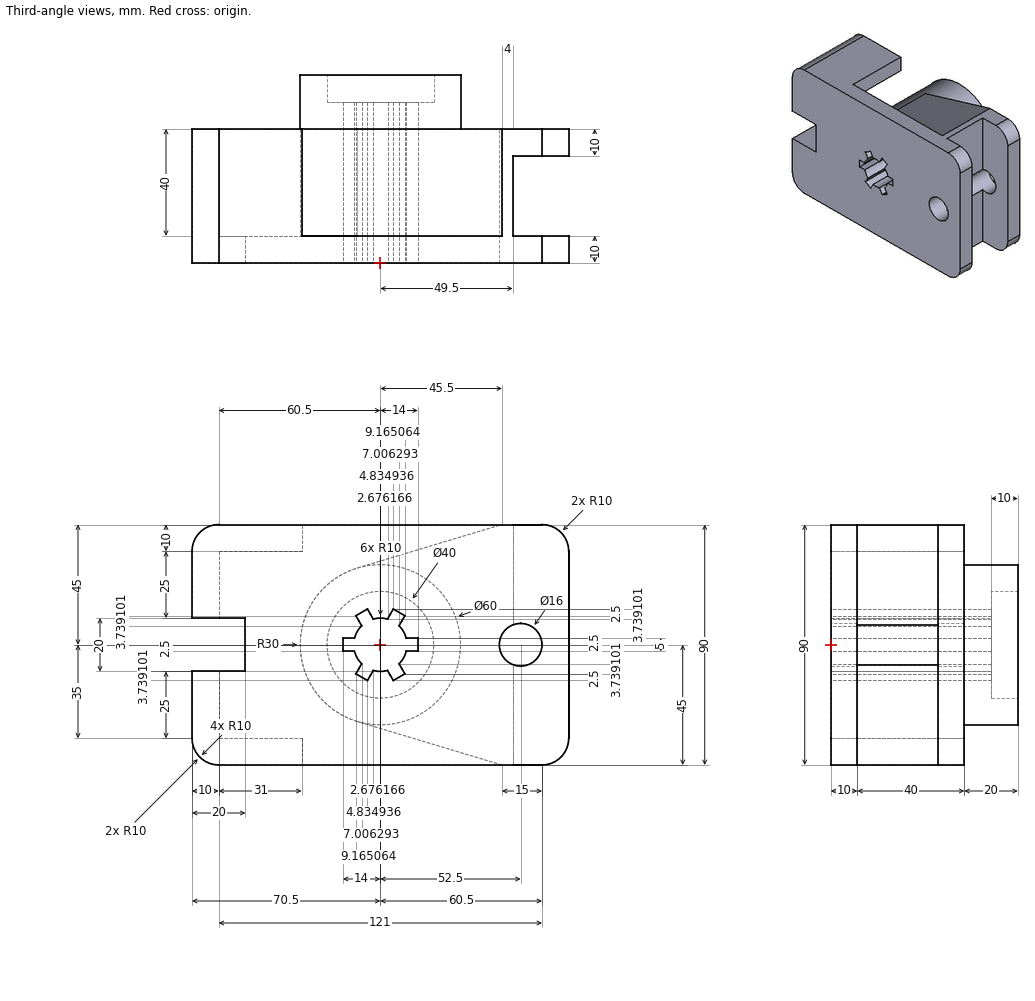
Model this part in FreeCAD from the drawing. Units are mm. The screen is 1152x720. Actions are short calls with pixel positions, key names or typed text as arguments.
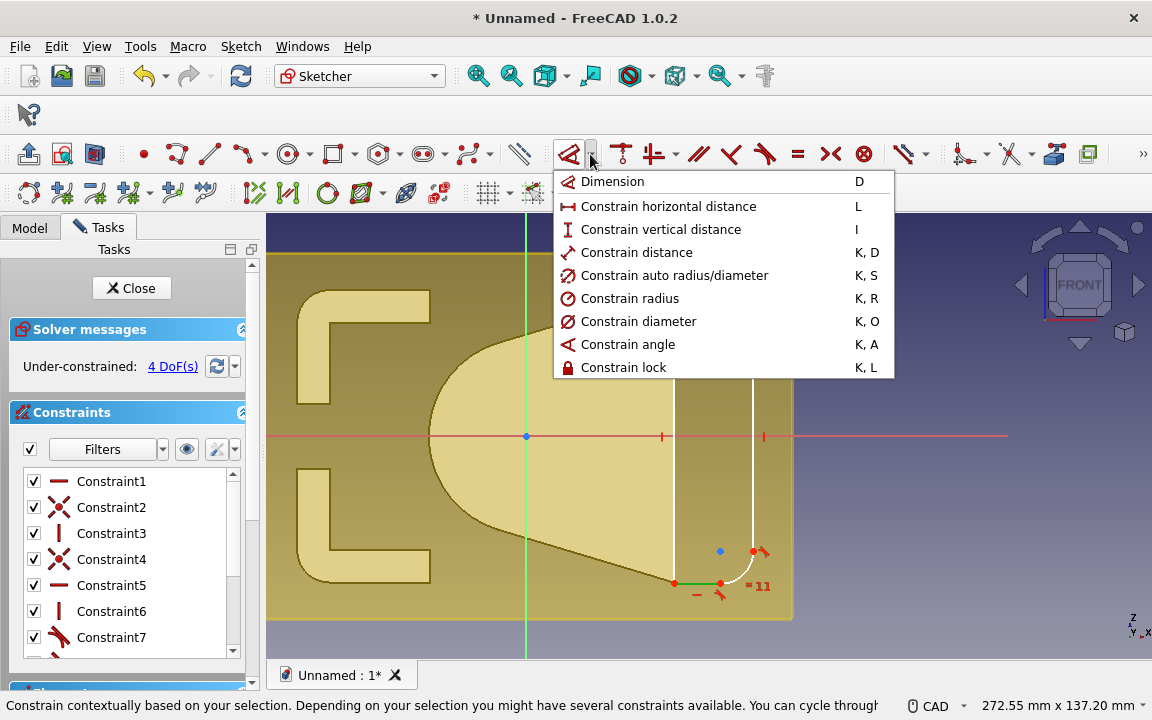
click(724, 206)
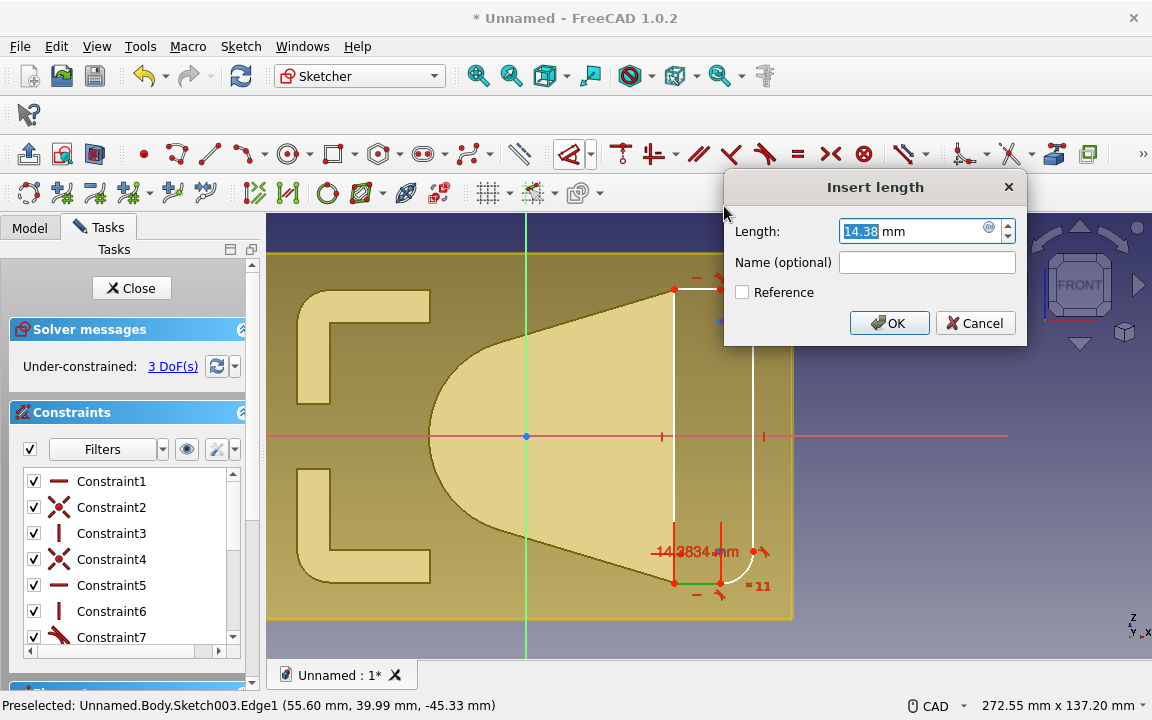
text(15)
key(Return)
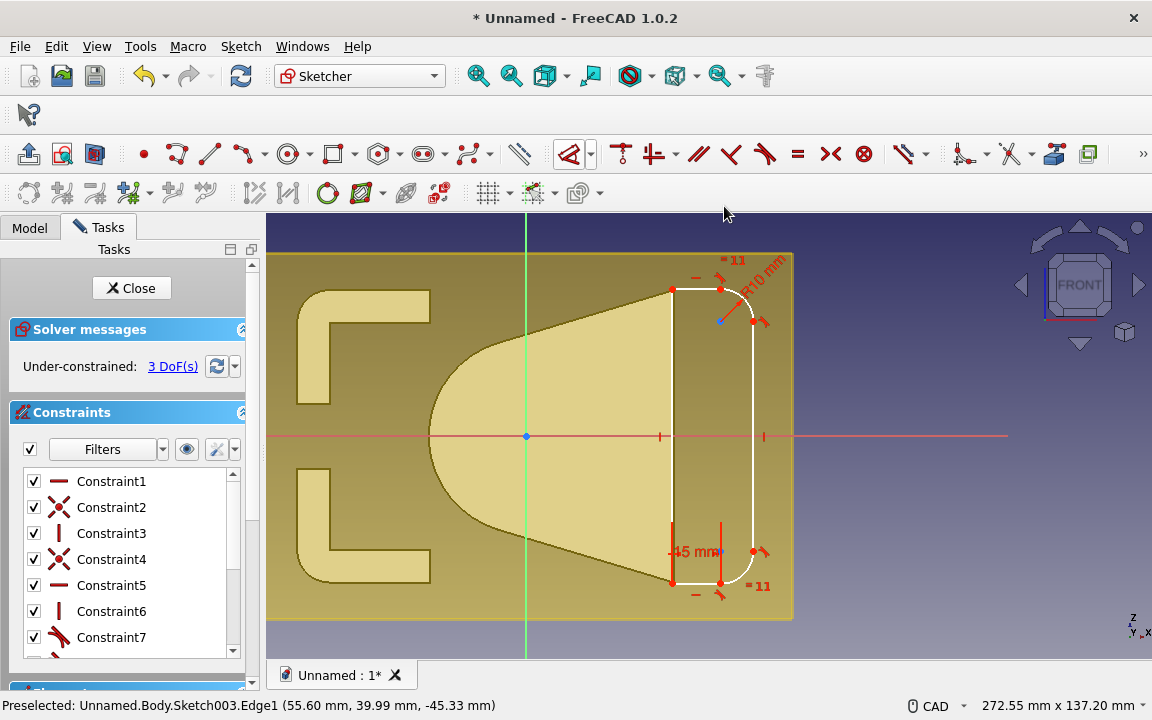
click(672, 495)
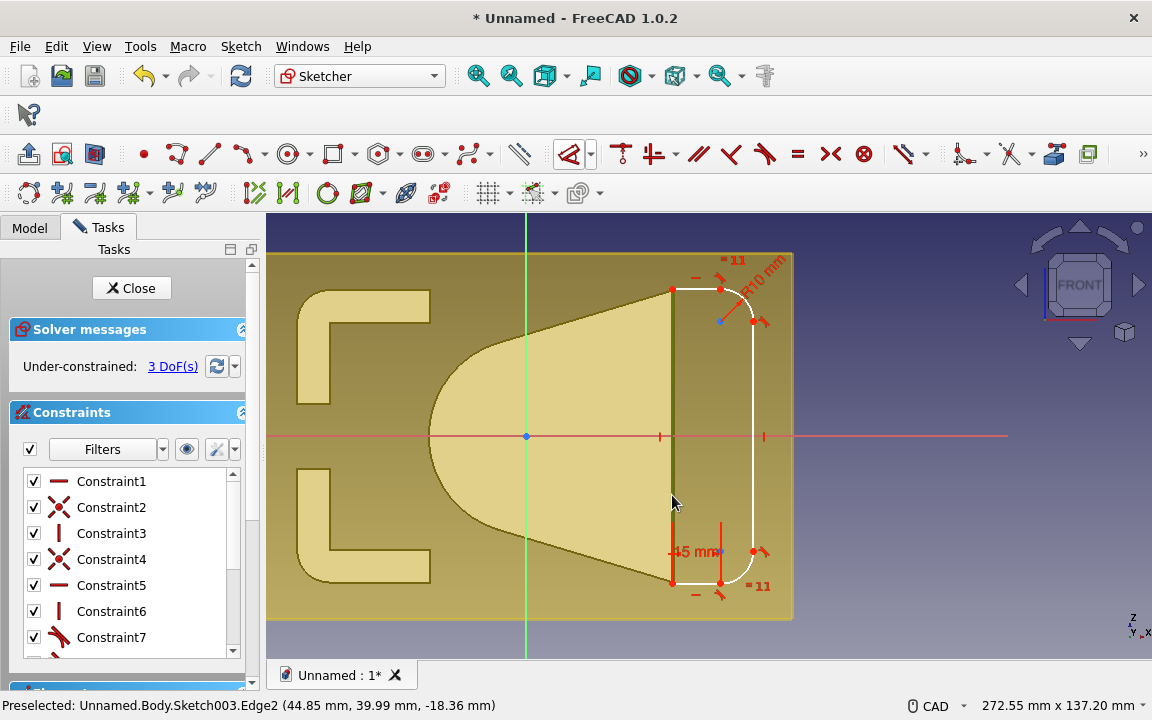
key(i)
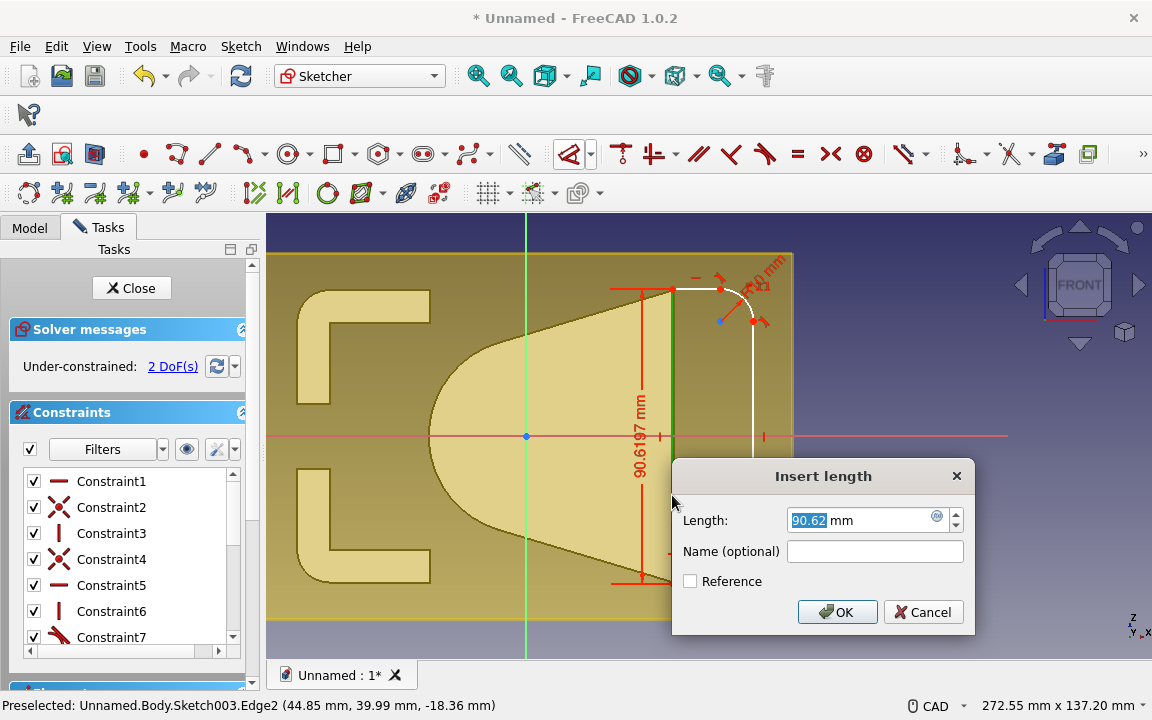
text(90)
key(Return)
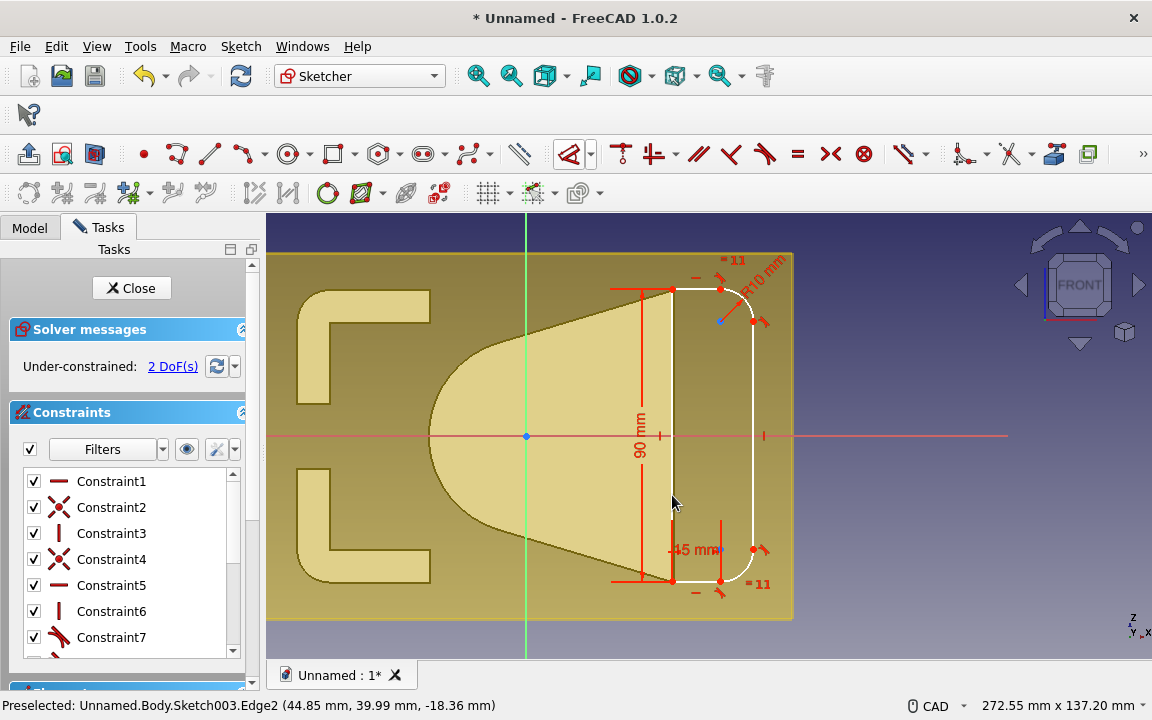
click(721, 582)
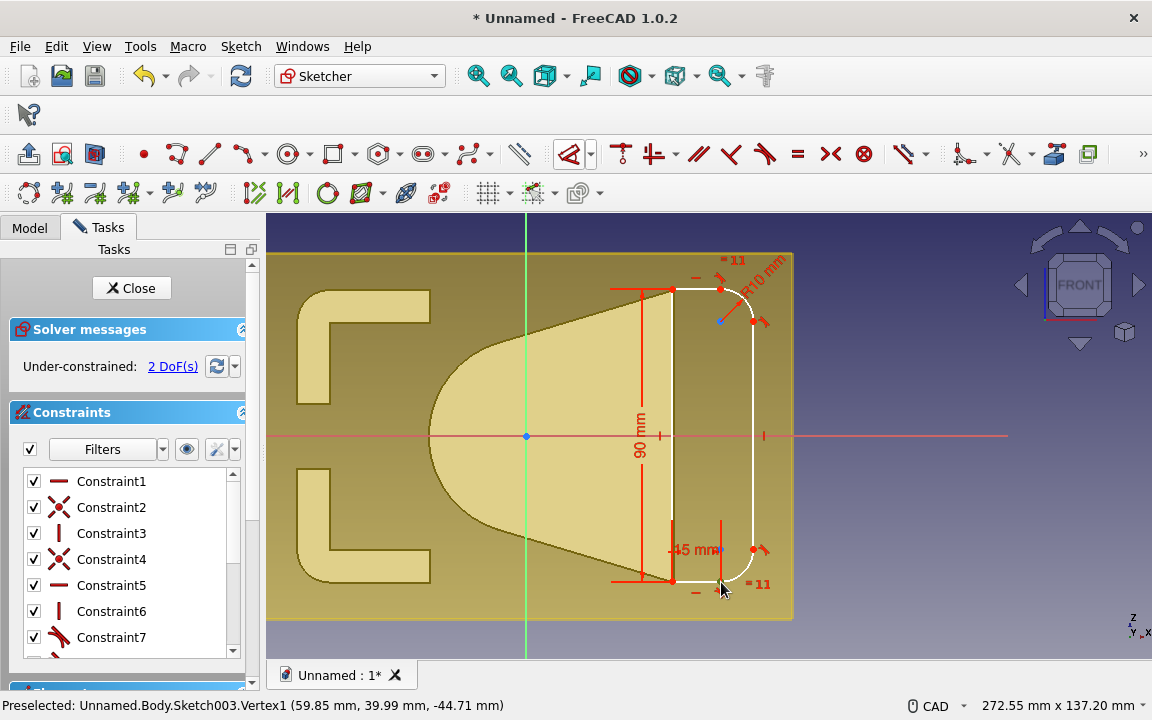
click(590, 154)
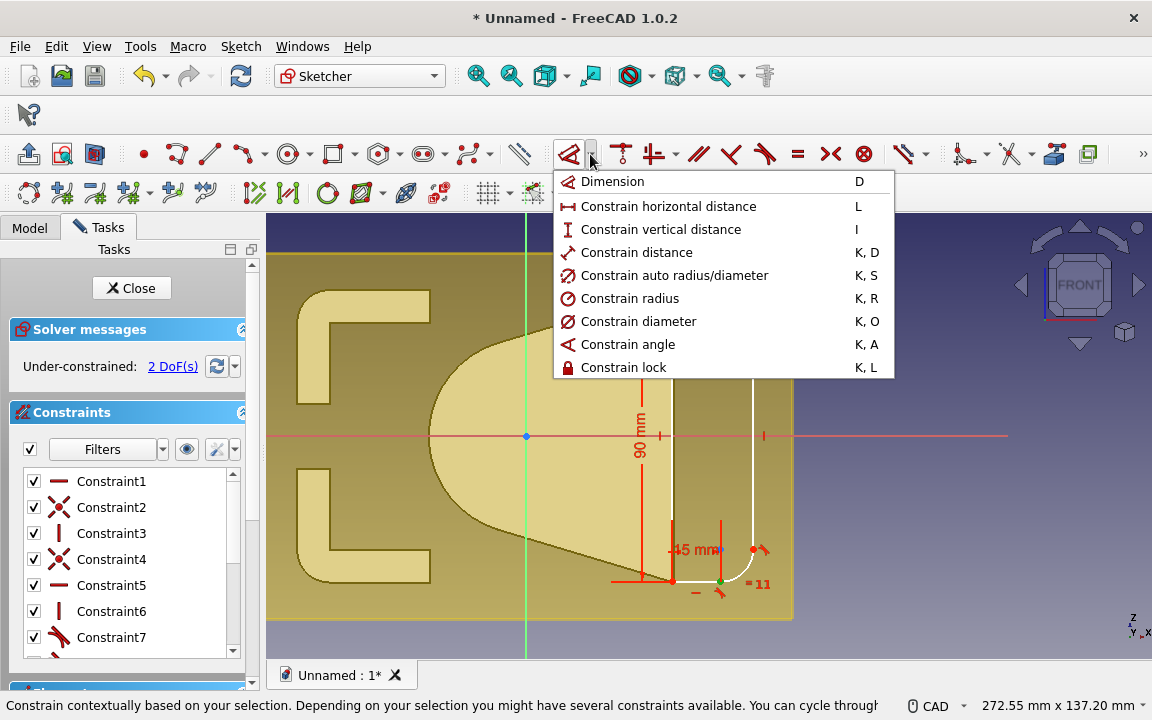
click(724, 230)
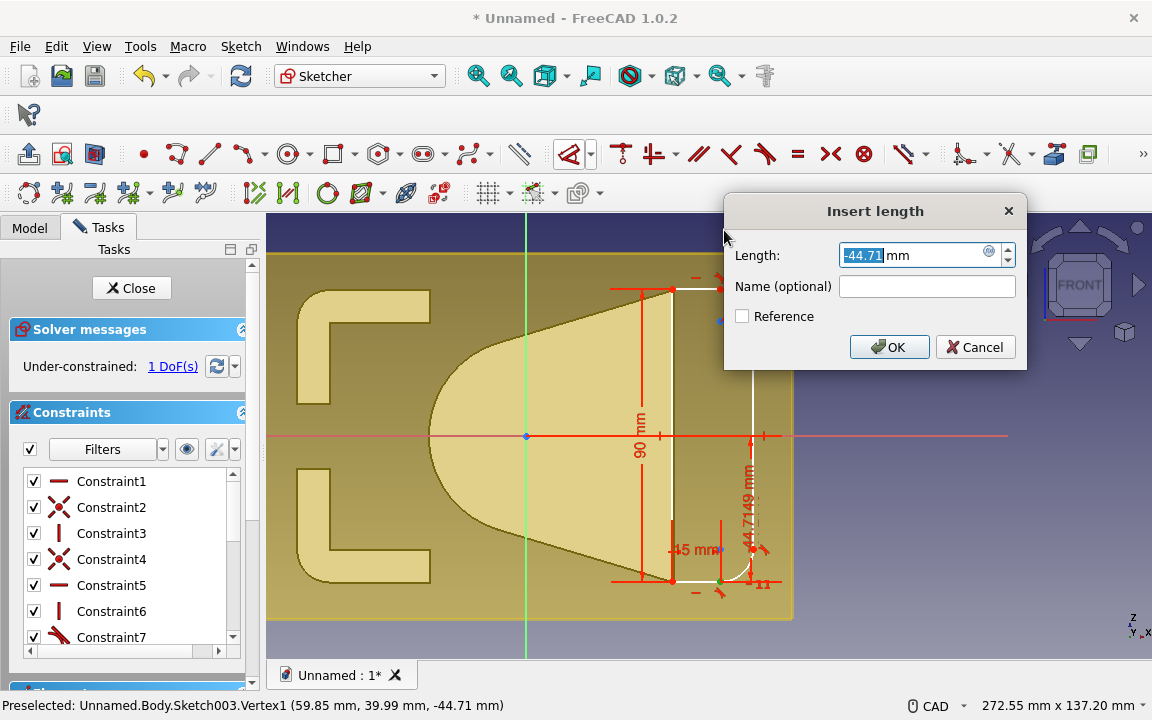
text(-45)
key(Return)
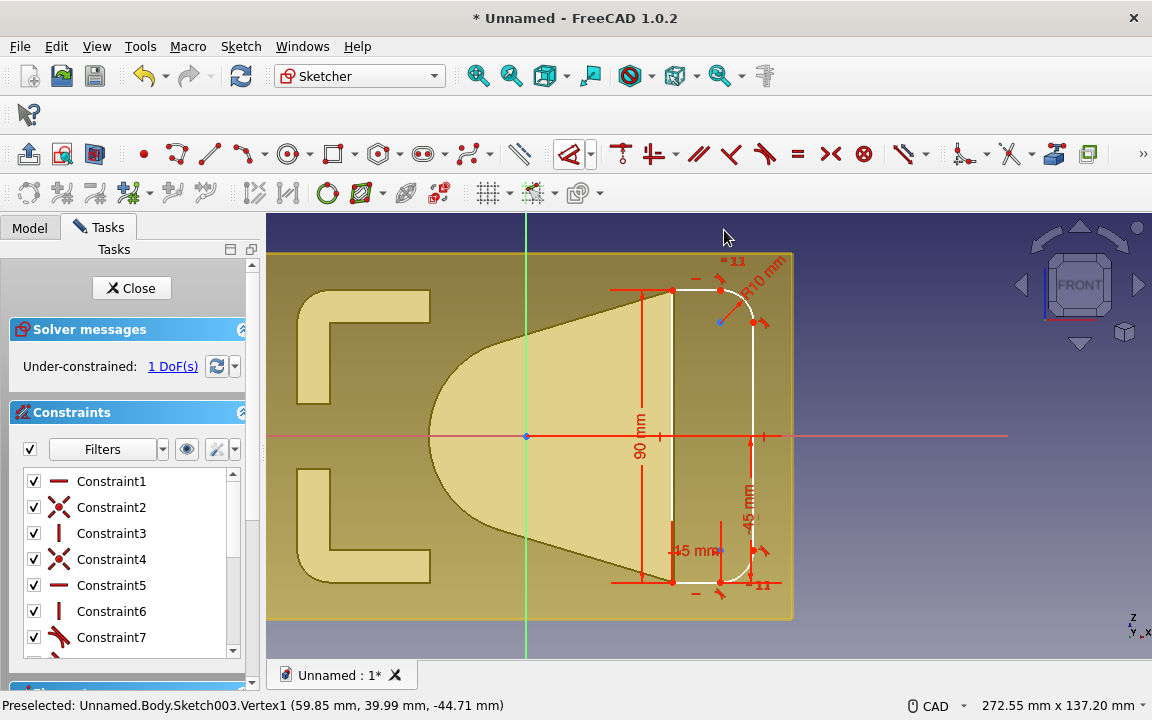
click(721, 583)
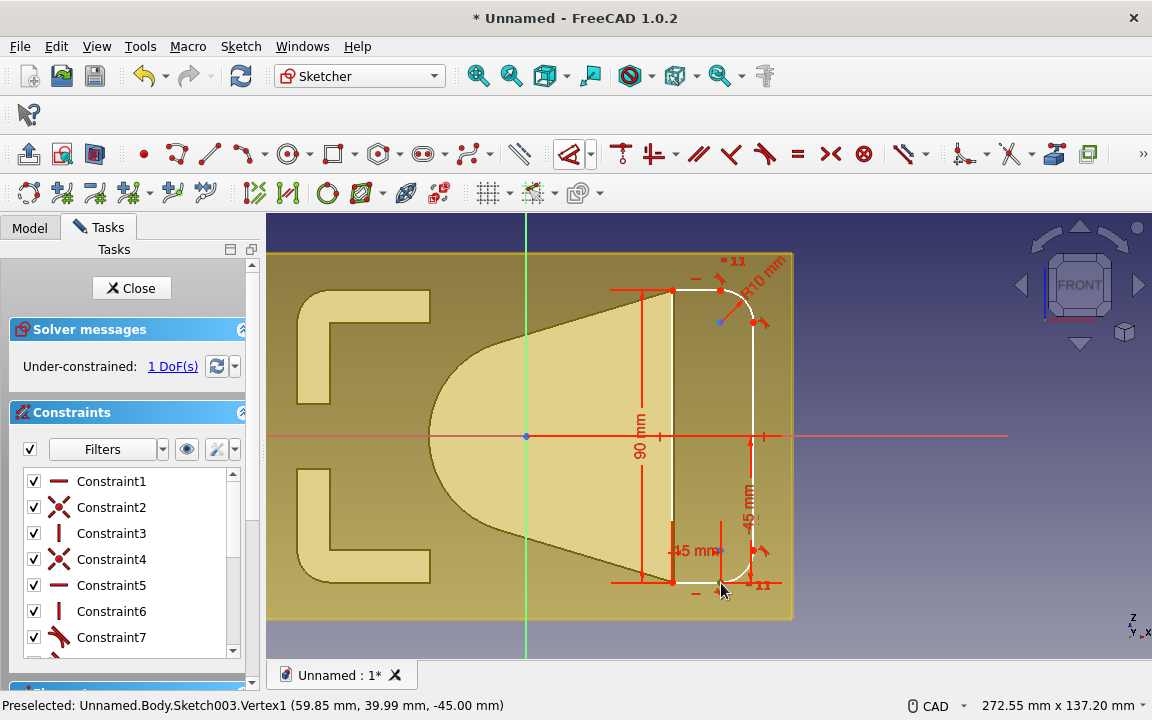
click(590, 154)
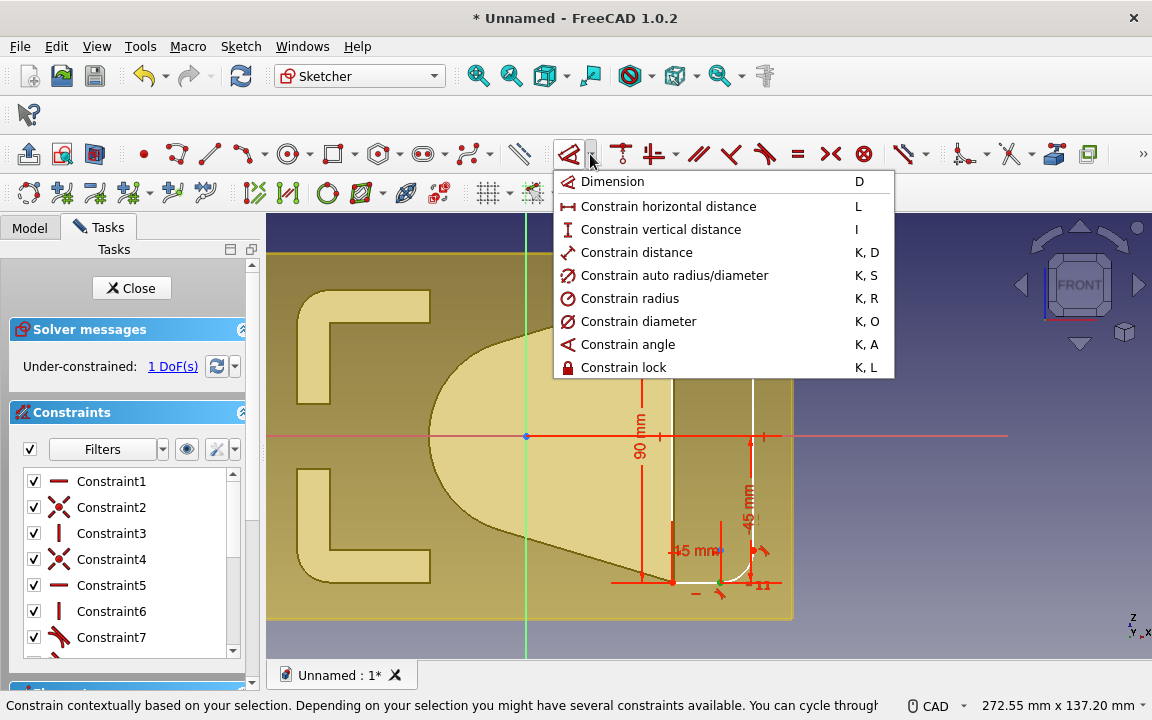
click(724, 206)